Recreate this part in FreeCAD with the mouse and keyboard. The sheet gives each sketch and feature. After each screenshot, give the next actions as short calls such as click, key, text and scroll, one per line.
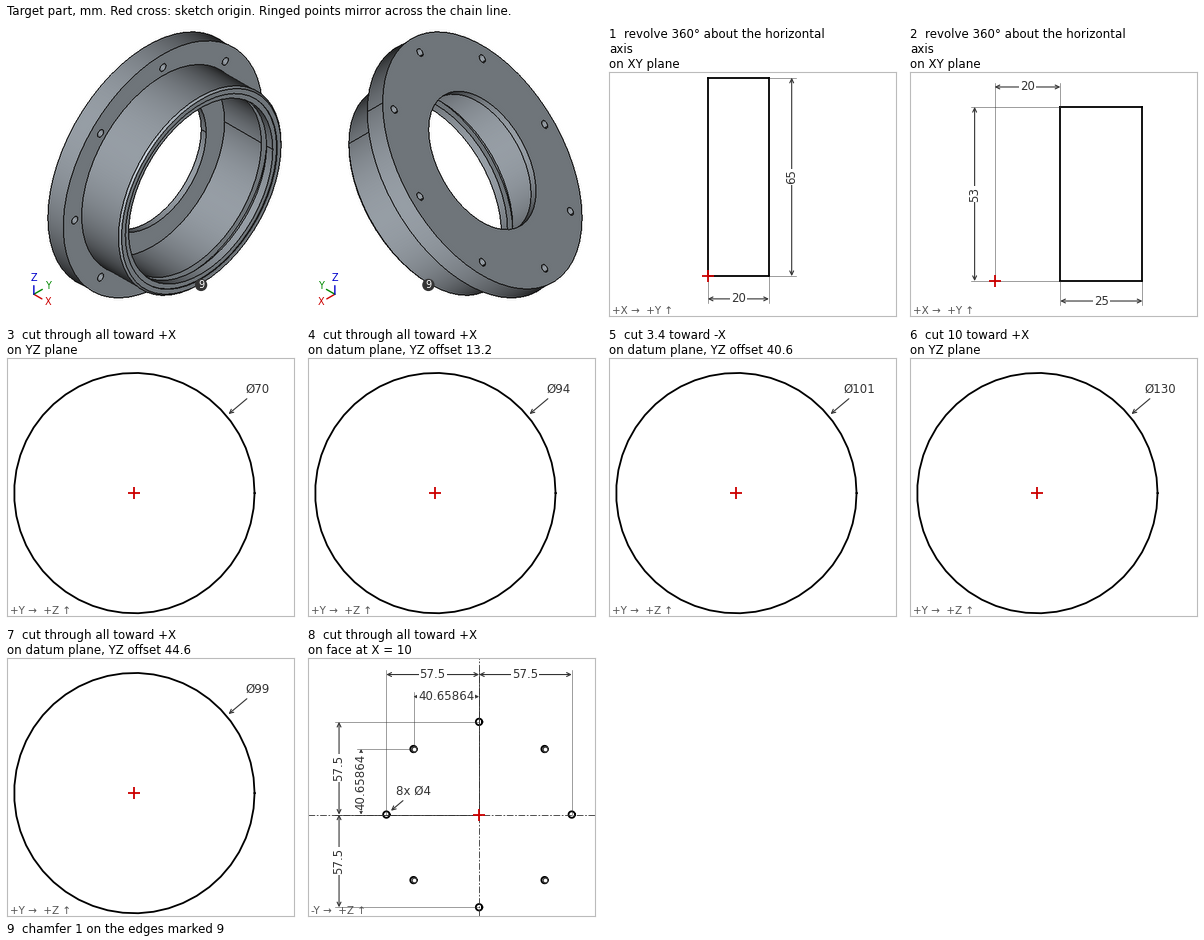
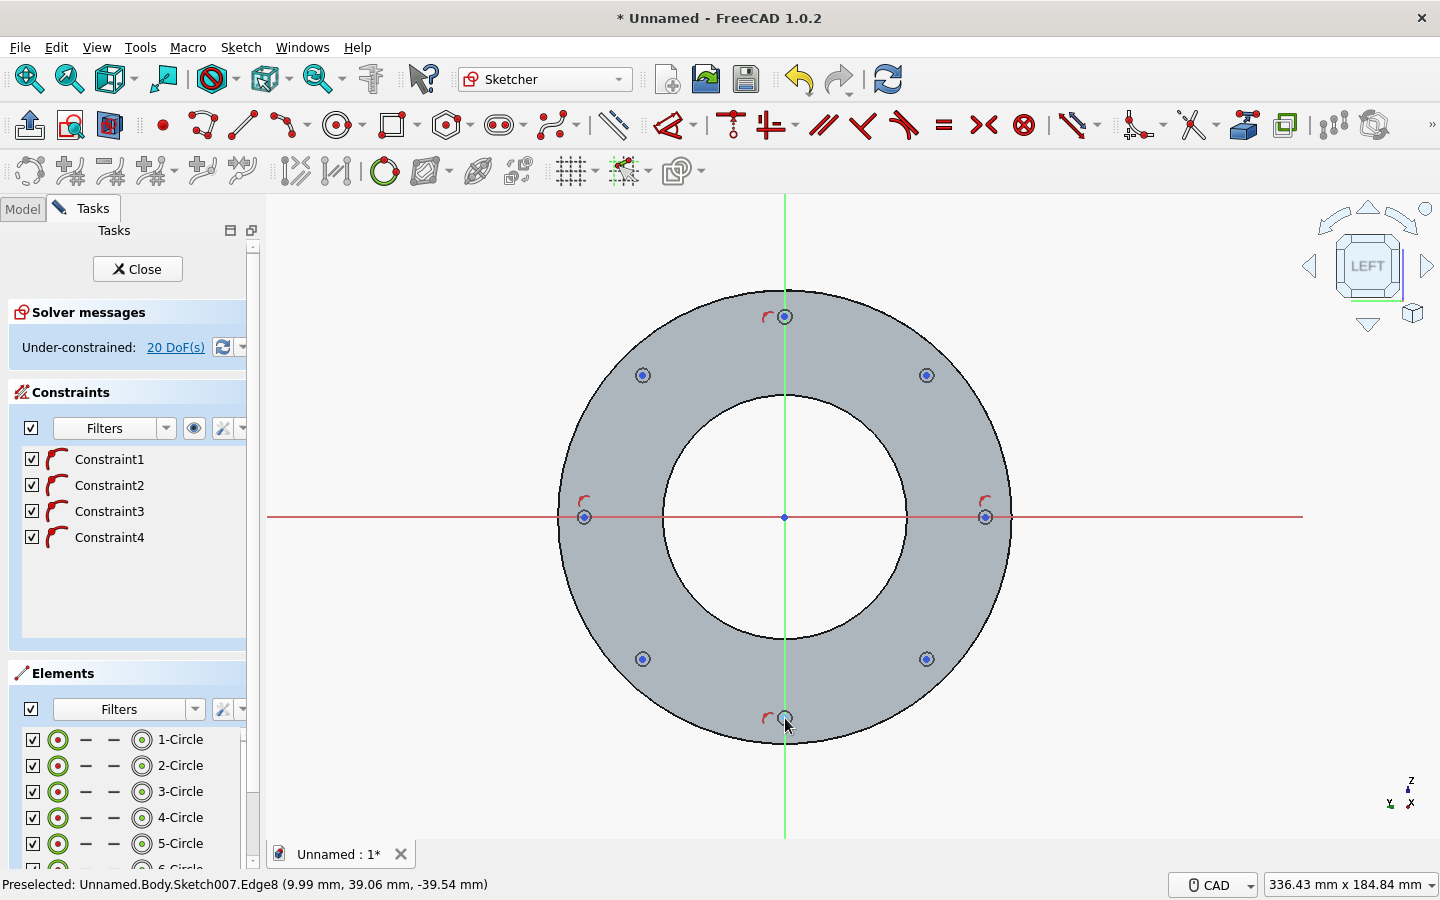
scroll(589, 512, up, 6)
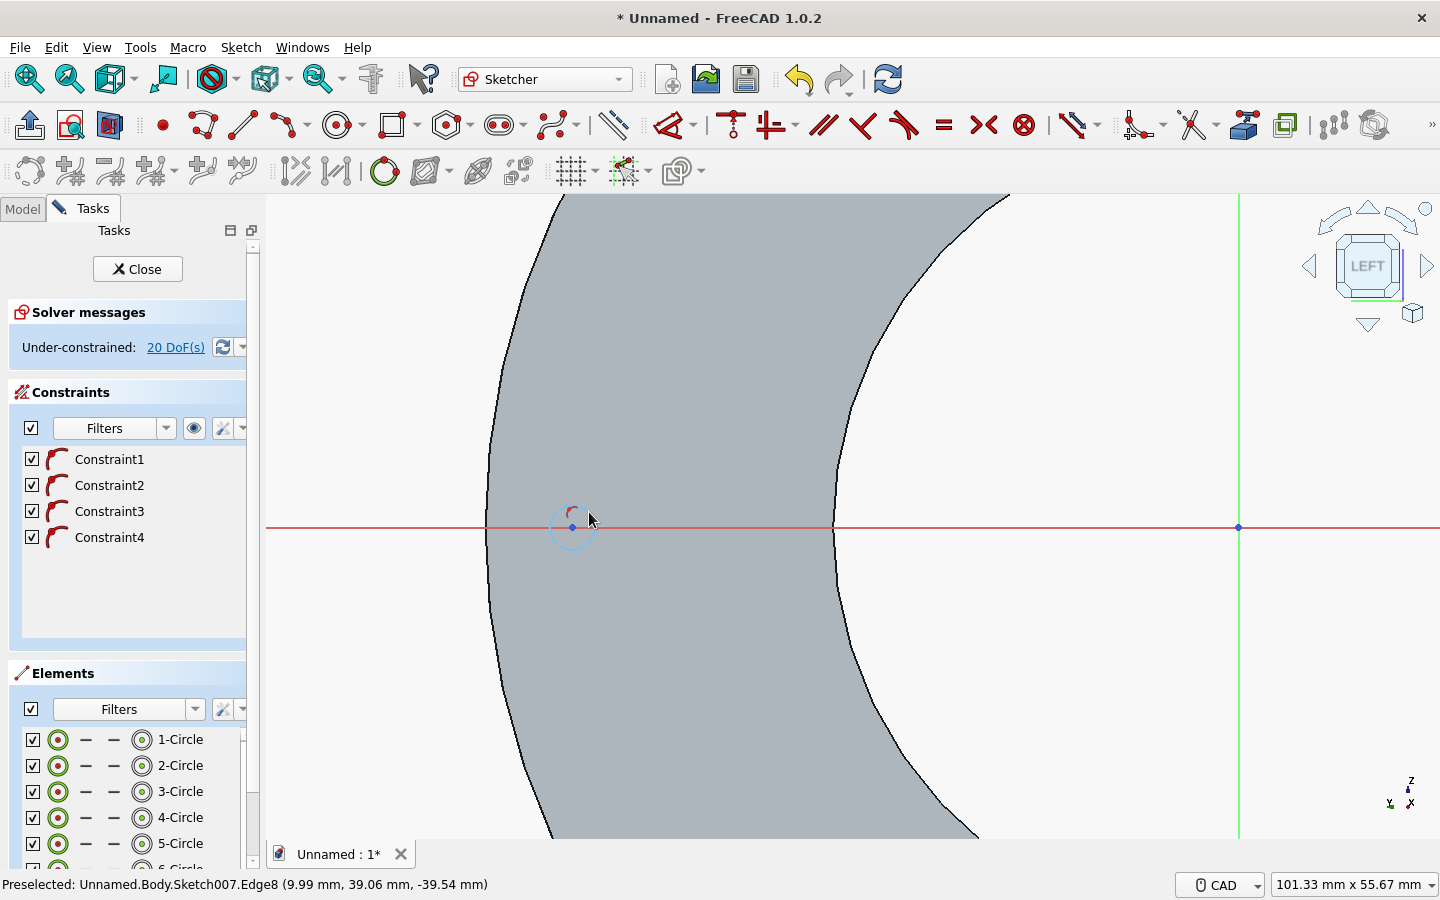
click(588, 512)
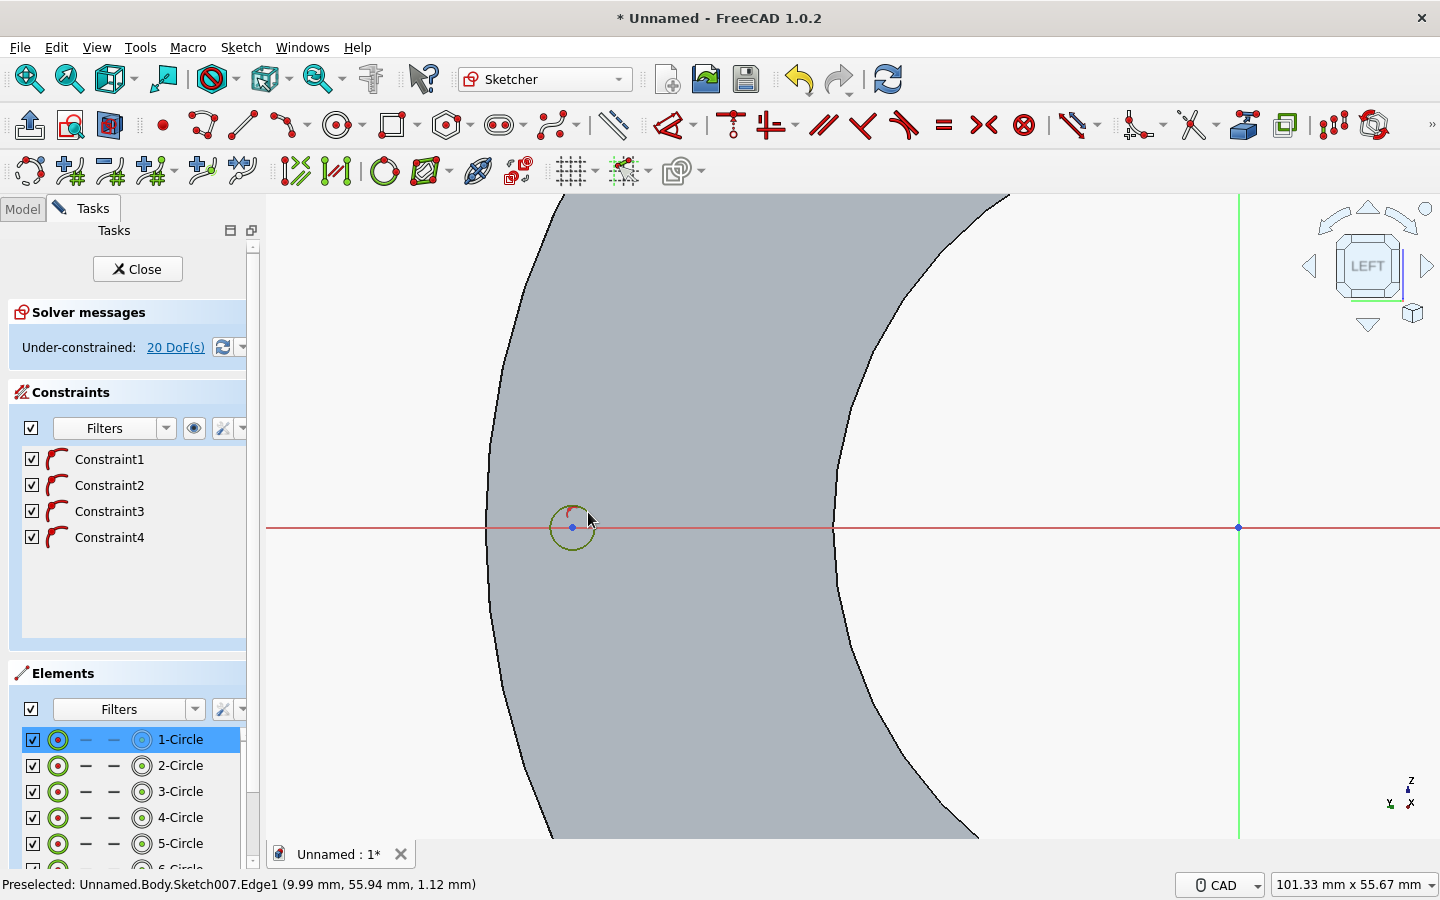
scroll(589, 512, down, 6)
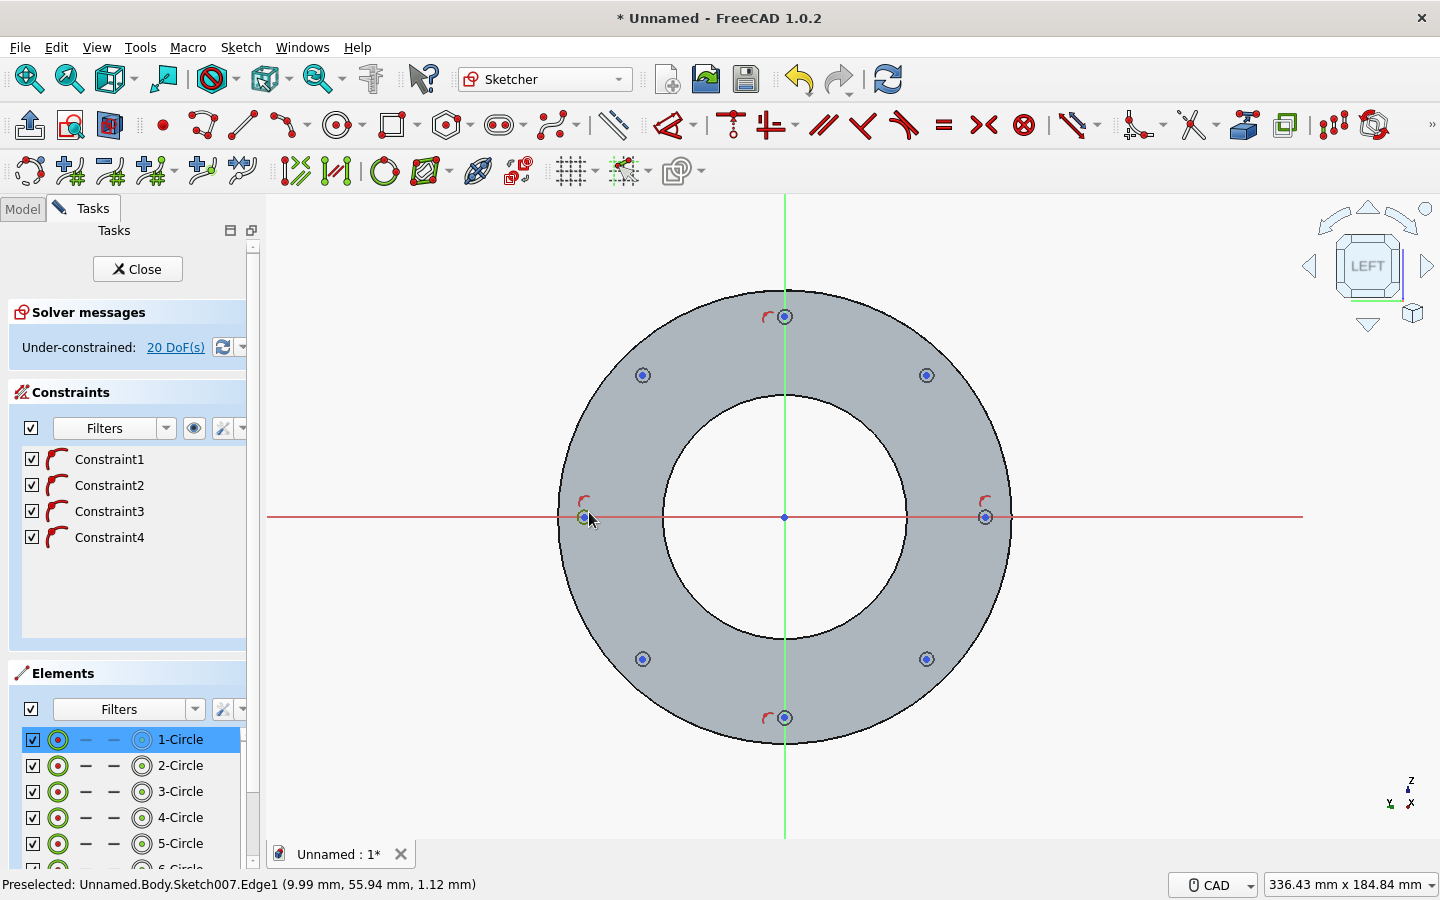
scroll(648, 371, up, 4)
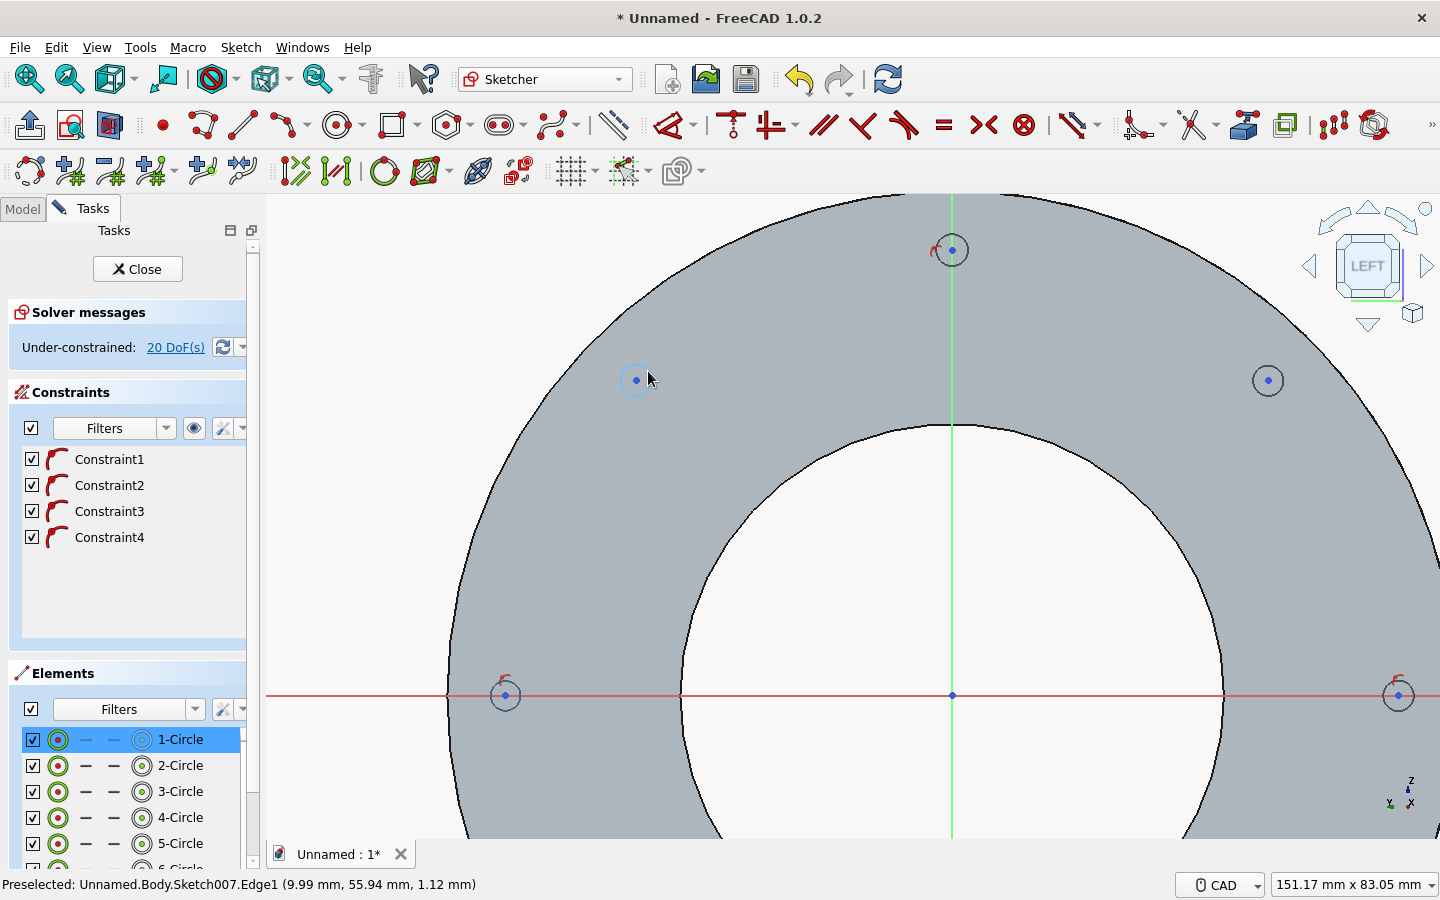
click(647, 370)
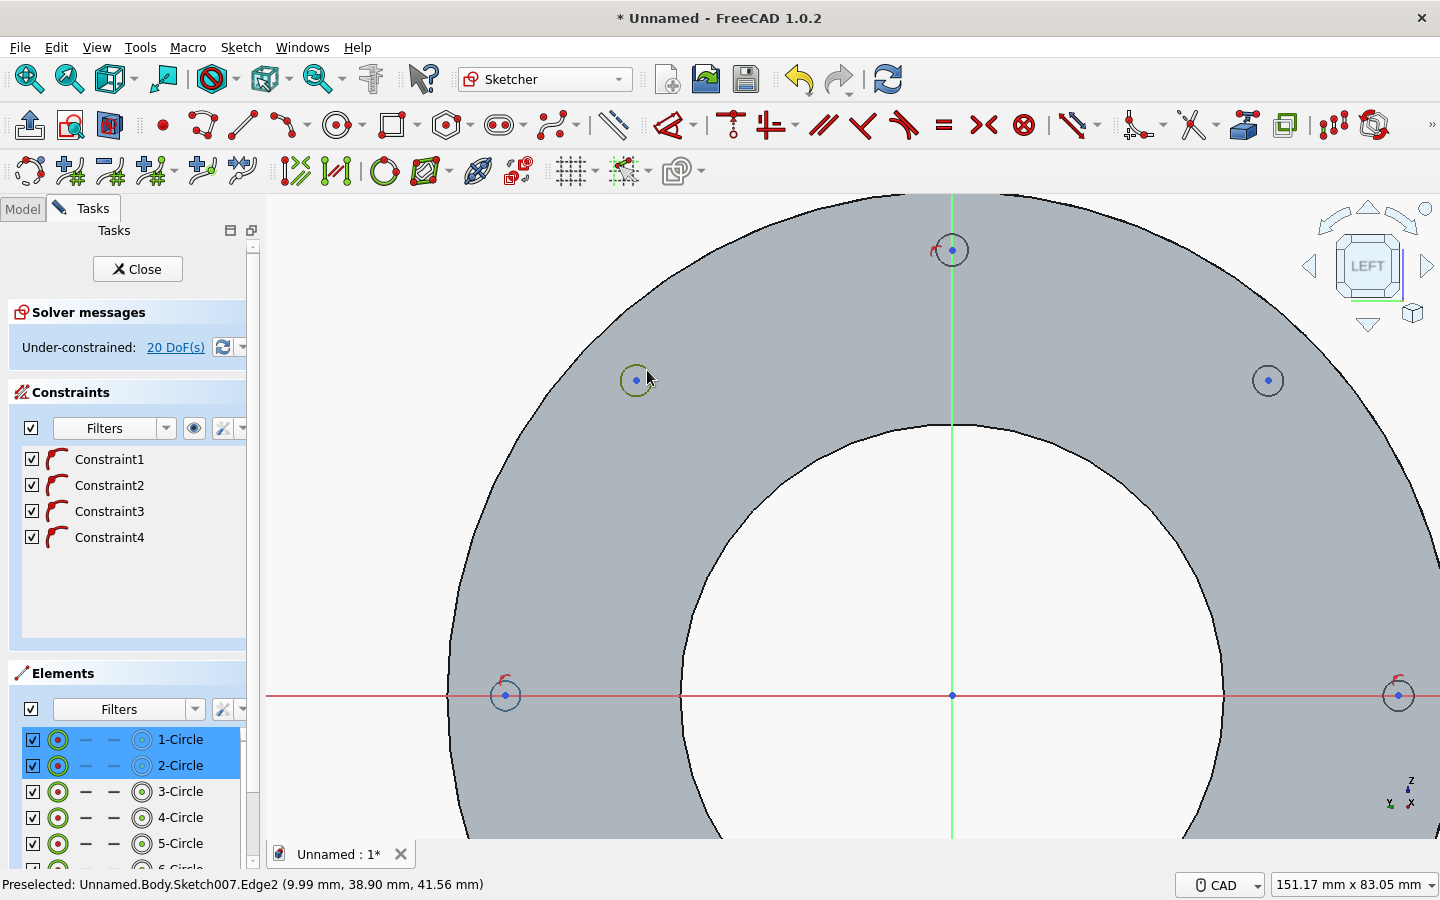
scroll(963, 239, up, 2)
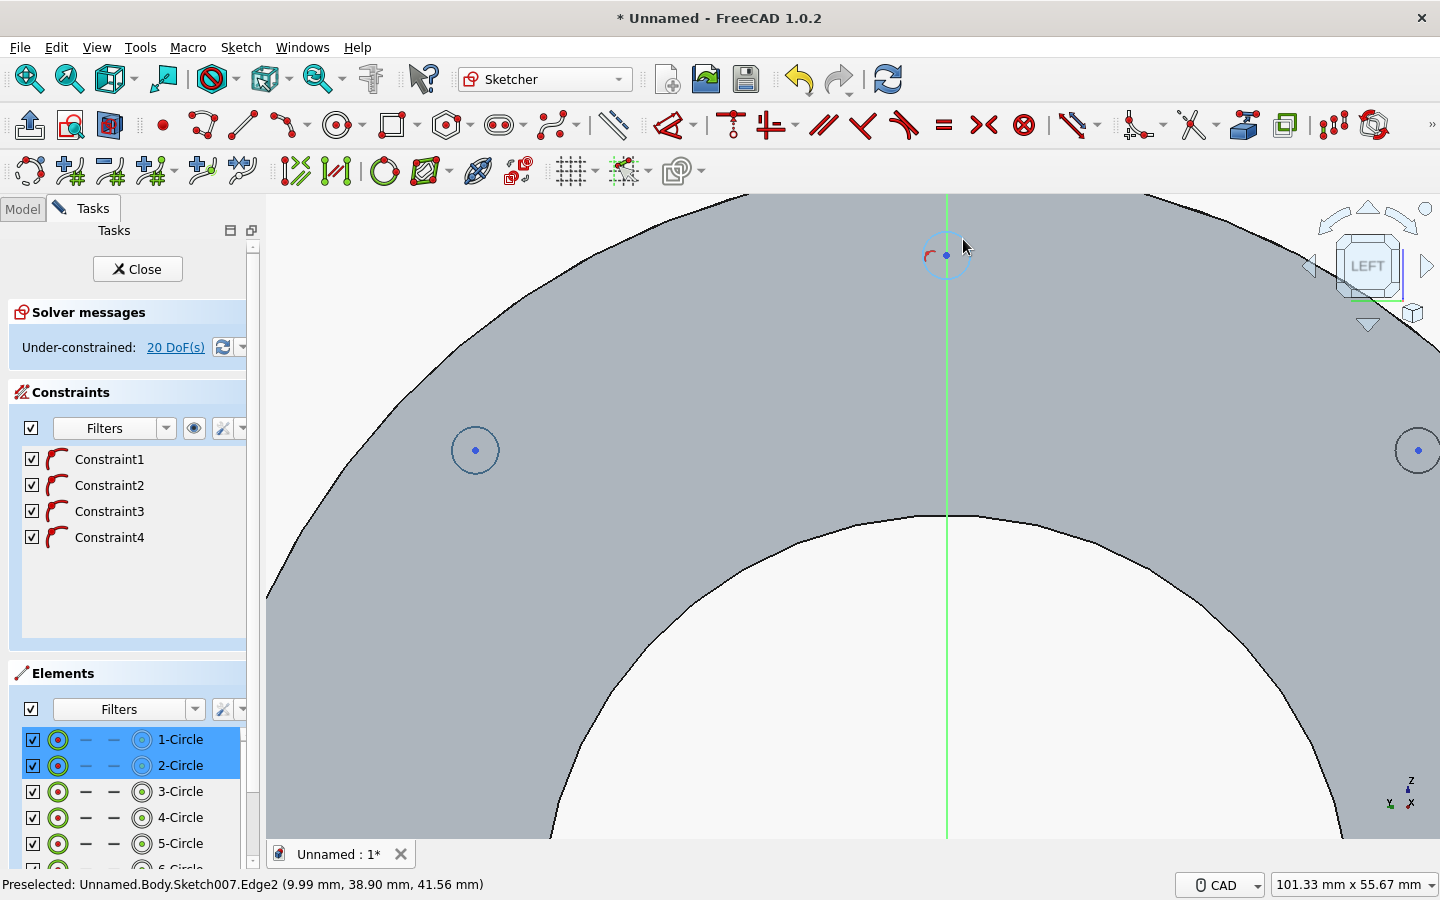
click(963, 239)